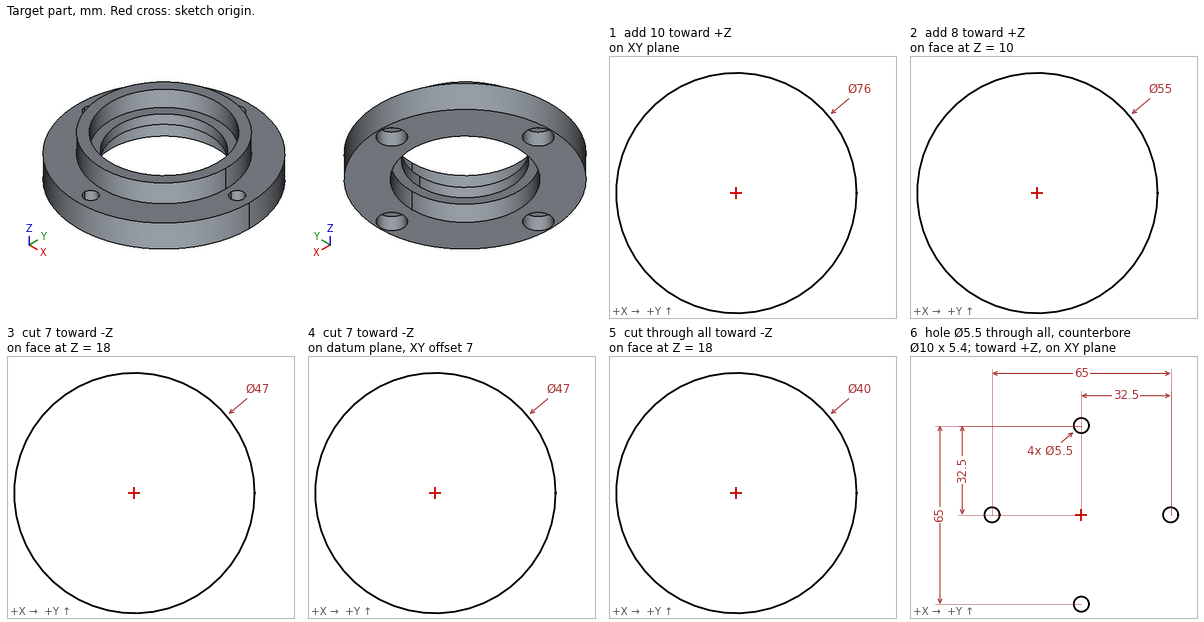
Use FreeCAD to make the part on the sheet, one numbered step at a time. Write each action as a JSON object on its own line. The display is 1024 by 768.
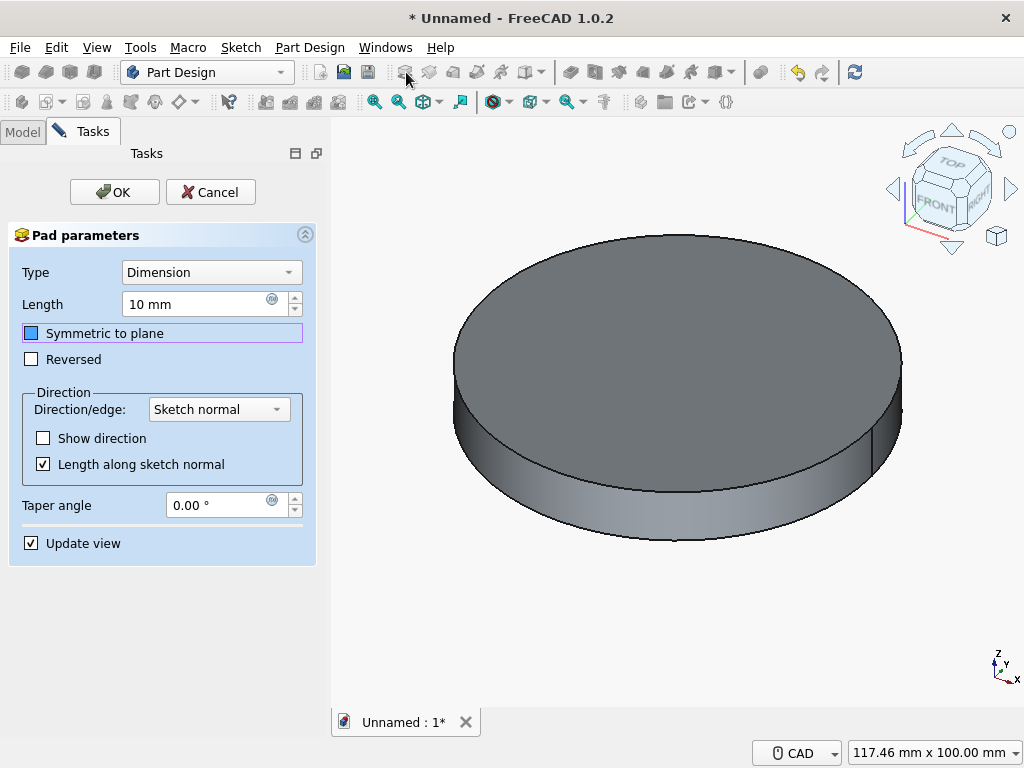
{"action": "left_click", "coordinate": [115, 192]}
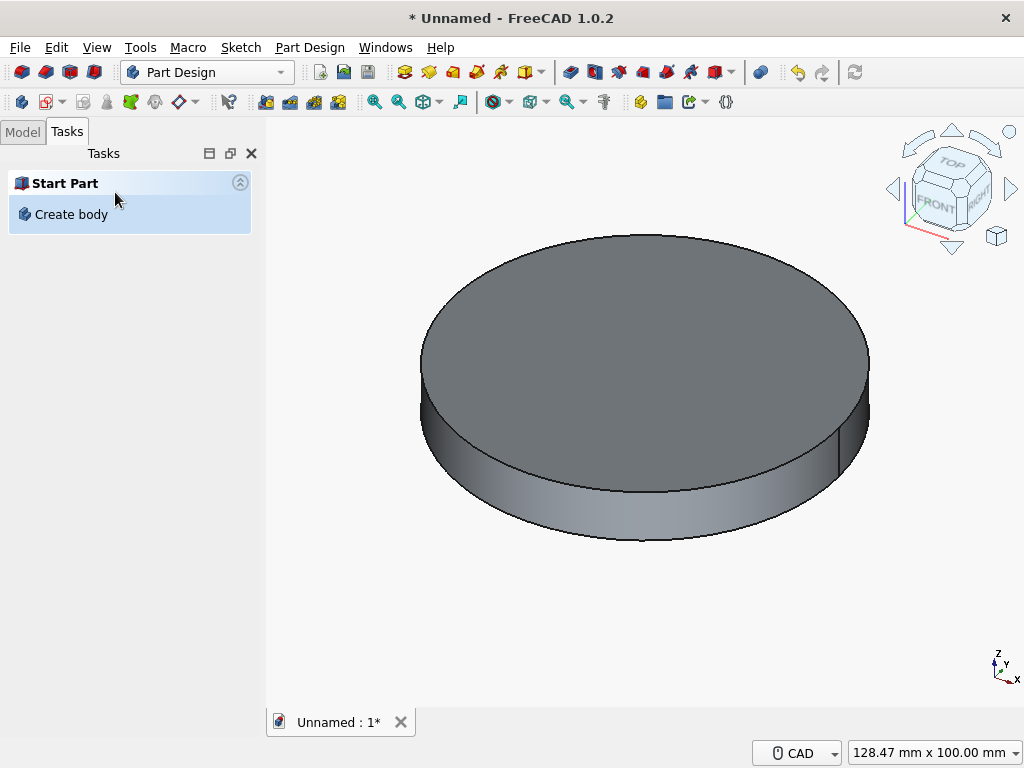
{"action": "left_click", "coordinate": [645, 363]}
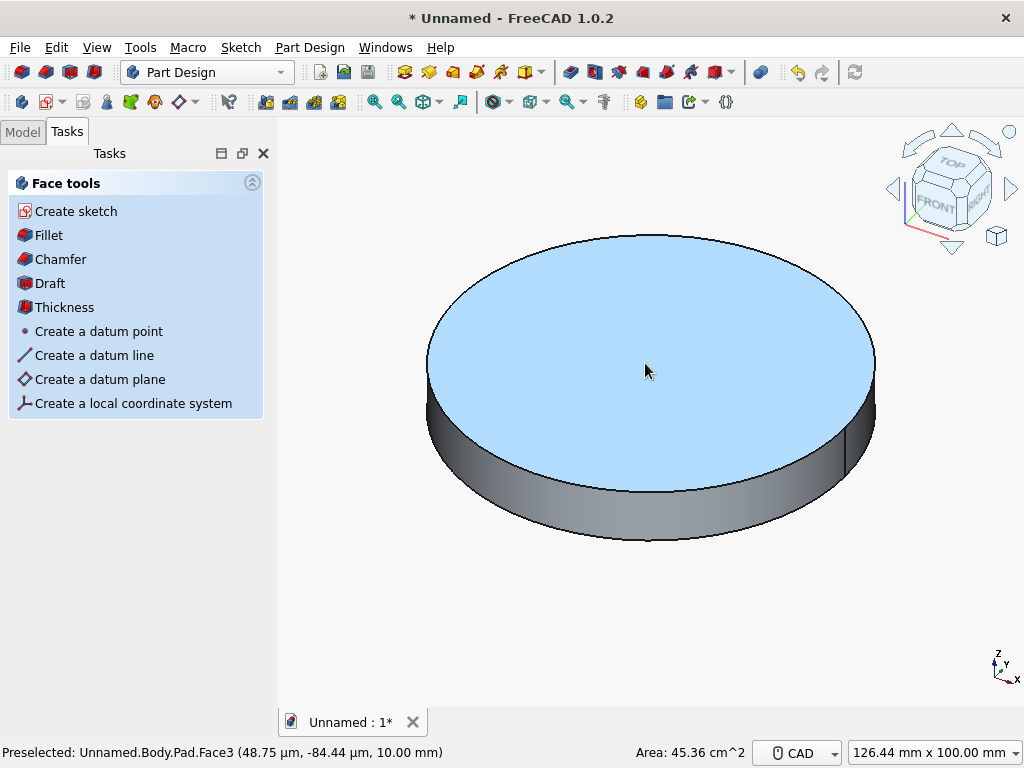
{"action": "left_click", "coordinate": [46, 102]}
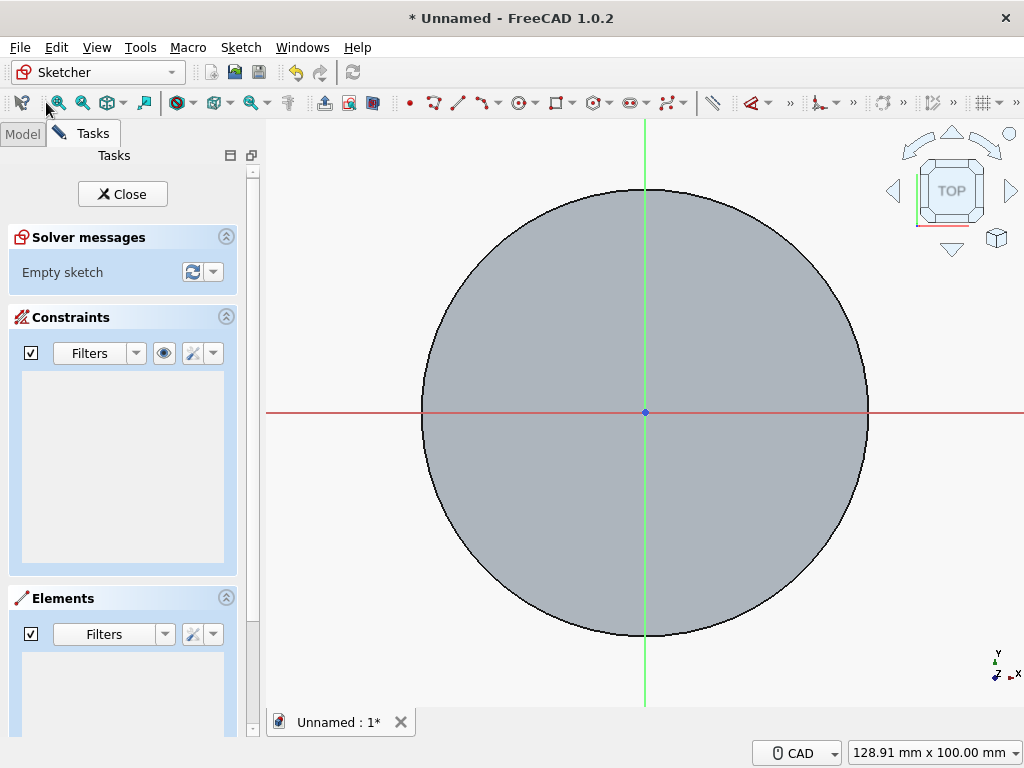
{"action": "key", "text": "g c"}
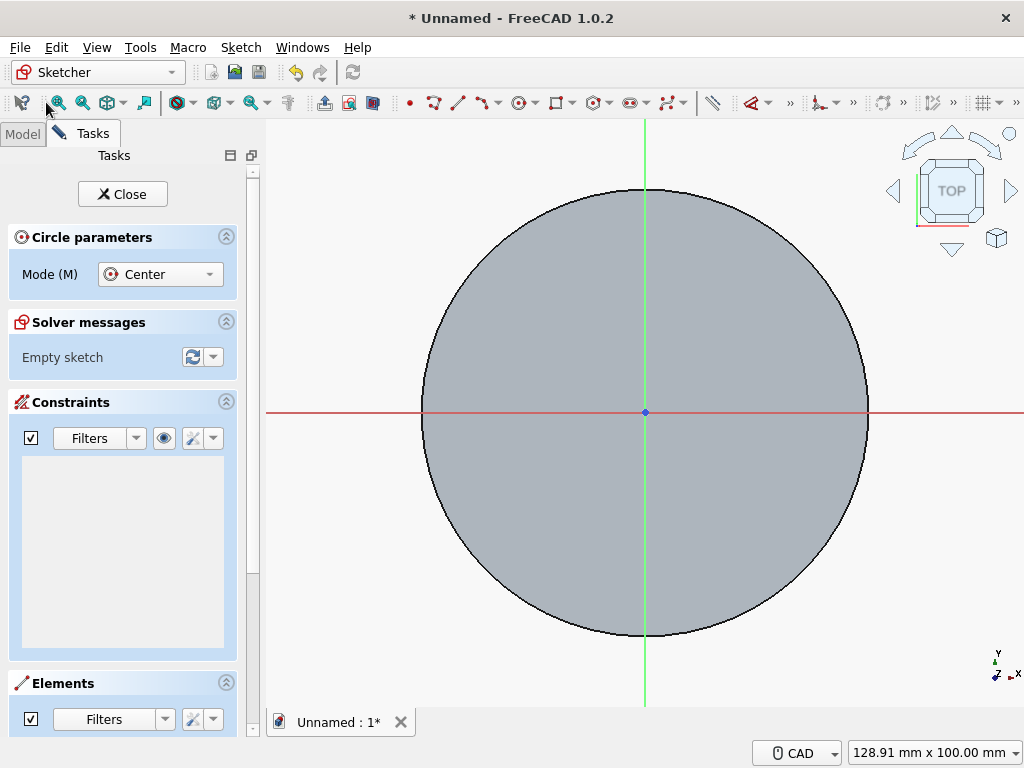
{"action": "left_click", "coordinate": [645, 413]}
{"action": "left_click", "coordinate": [759, 299]}
{"action": "key", "text": "Escape"}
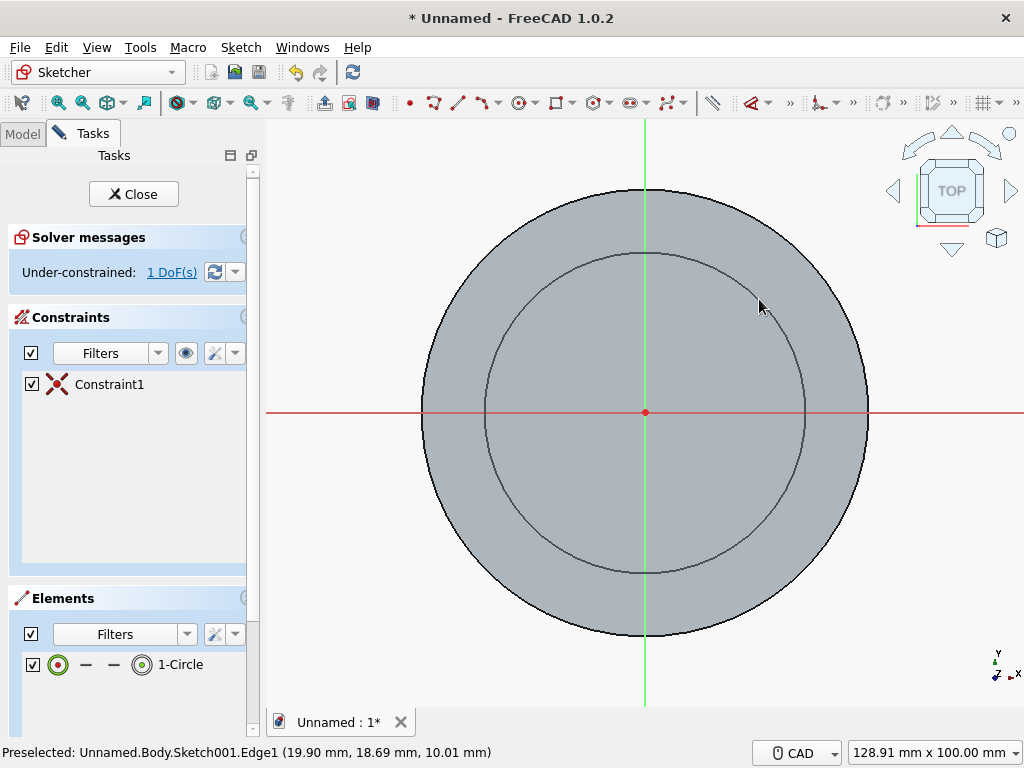
{"action": "left_click", "coordinate": [758, 299]}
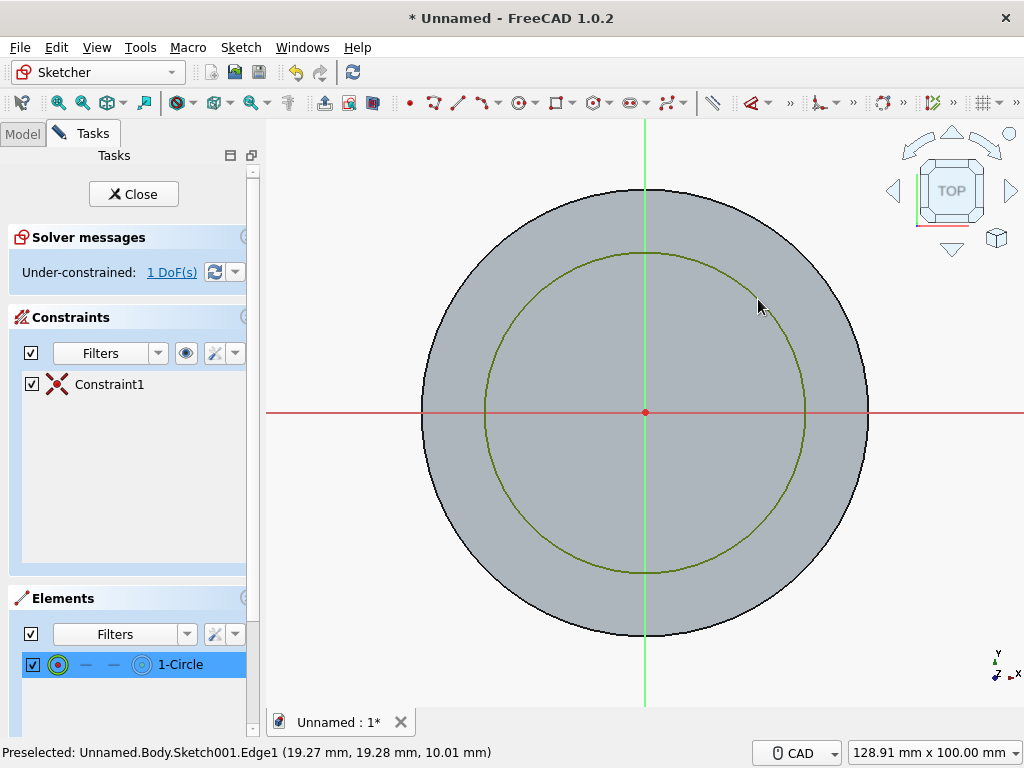
{"action": "key", "text": "k o"}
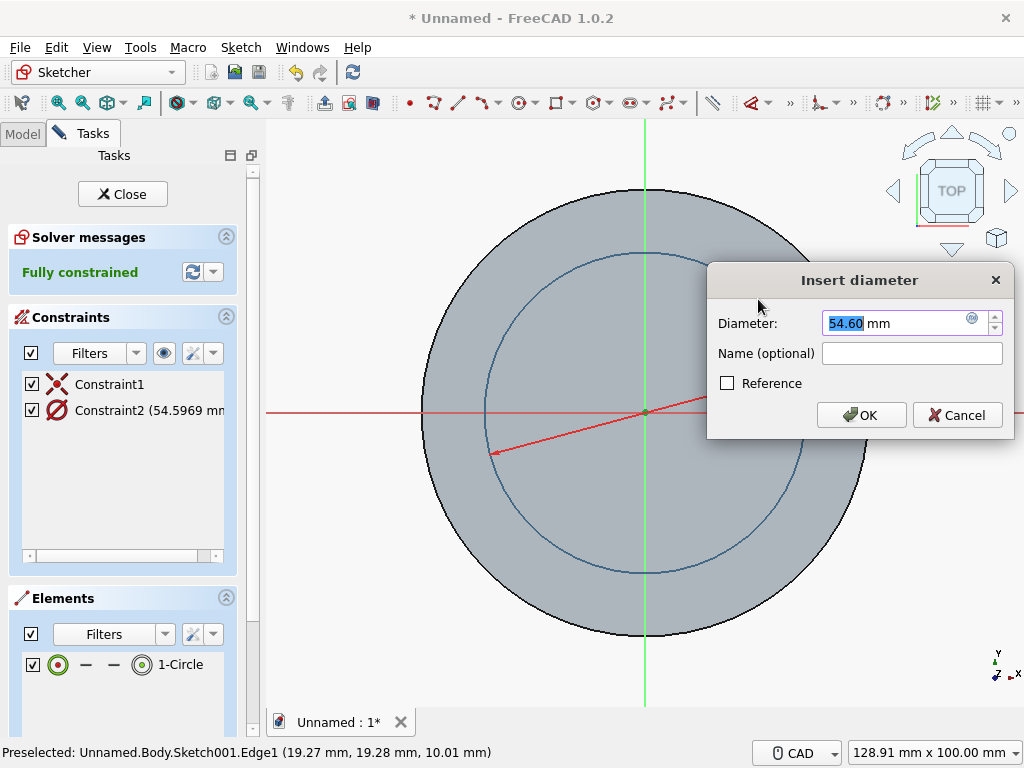
{"action": "type", "text": "55"}
{"action": "key", "text": "Return"}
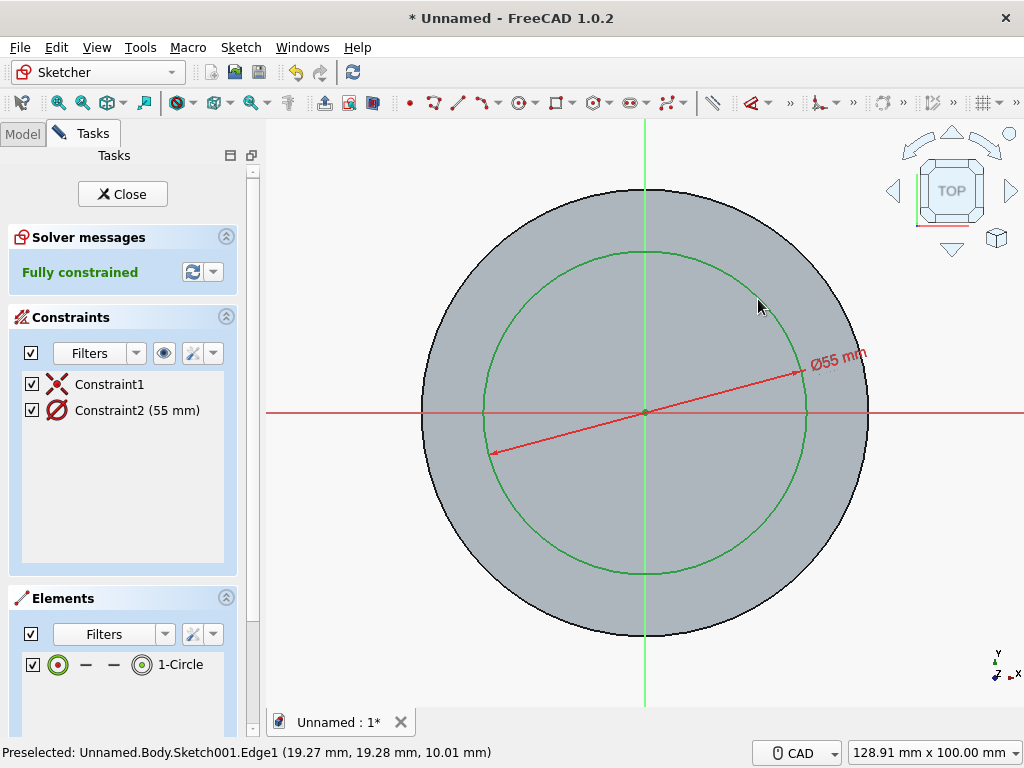
{"action": "left_click", "coordinate": [123, 194]}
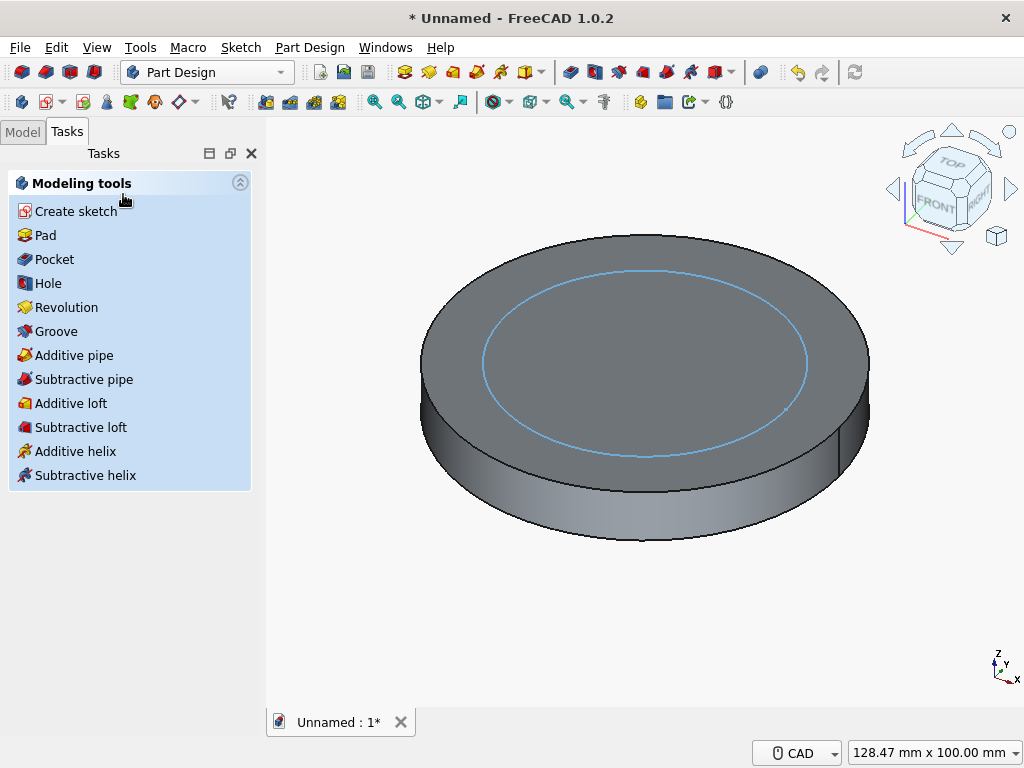
{"action": "left_click", "coordinate": [406, 72]}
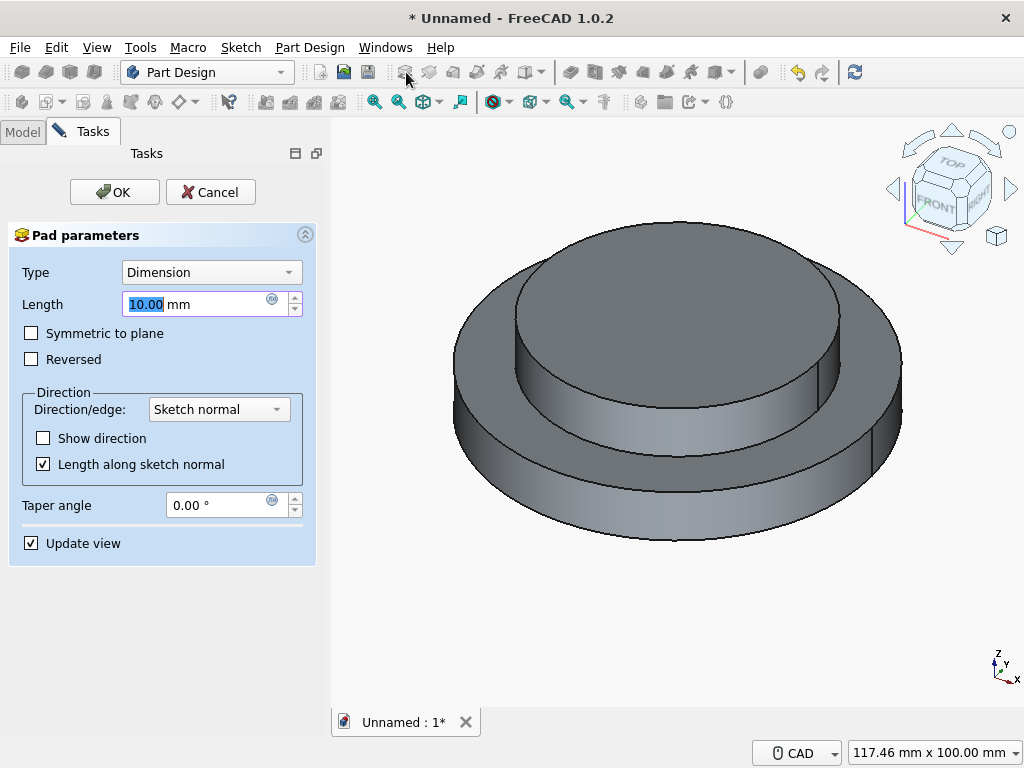
{"action": "type", "text": "8"}
{"action": "key", "text": "Tab"}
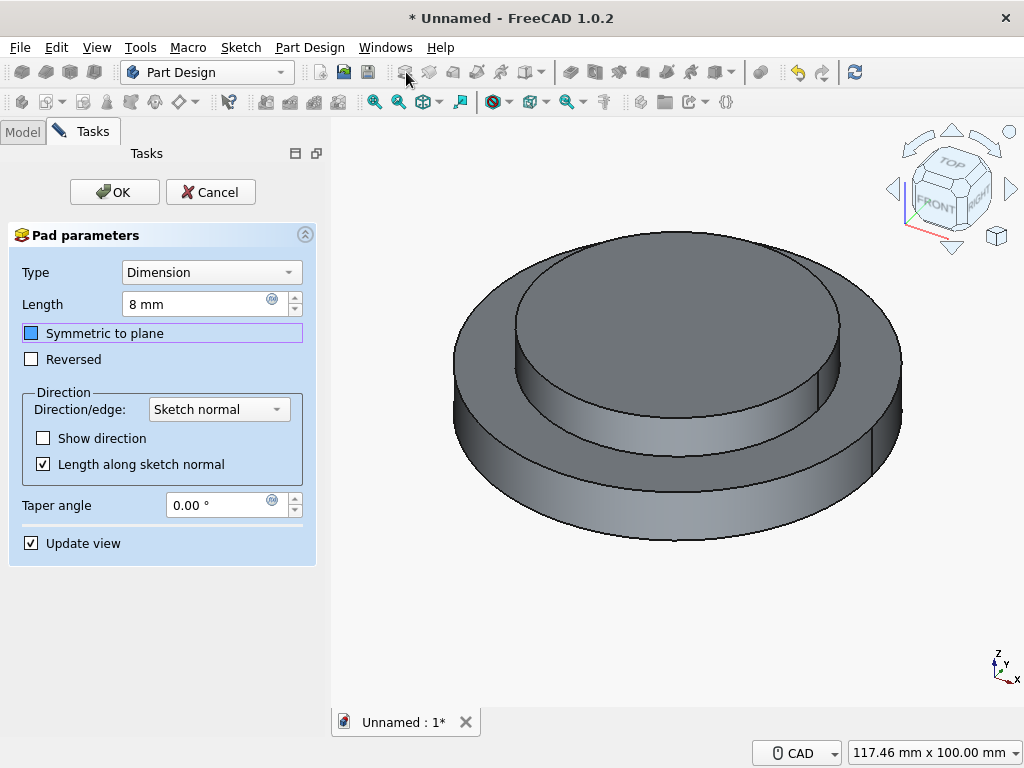
{"action": "left_click", "coordinate": [115, 192]}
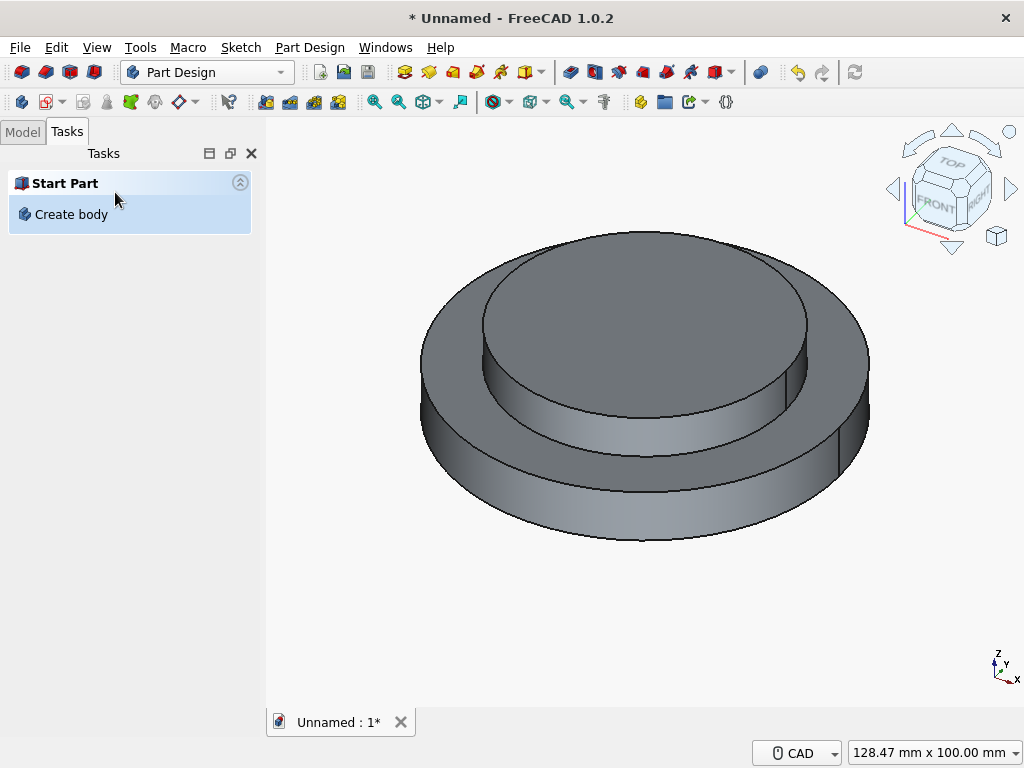
{"action": "left_click", "coordinate": [645, 324]}